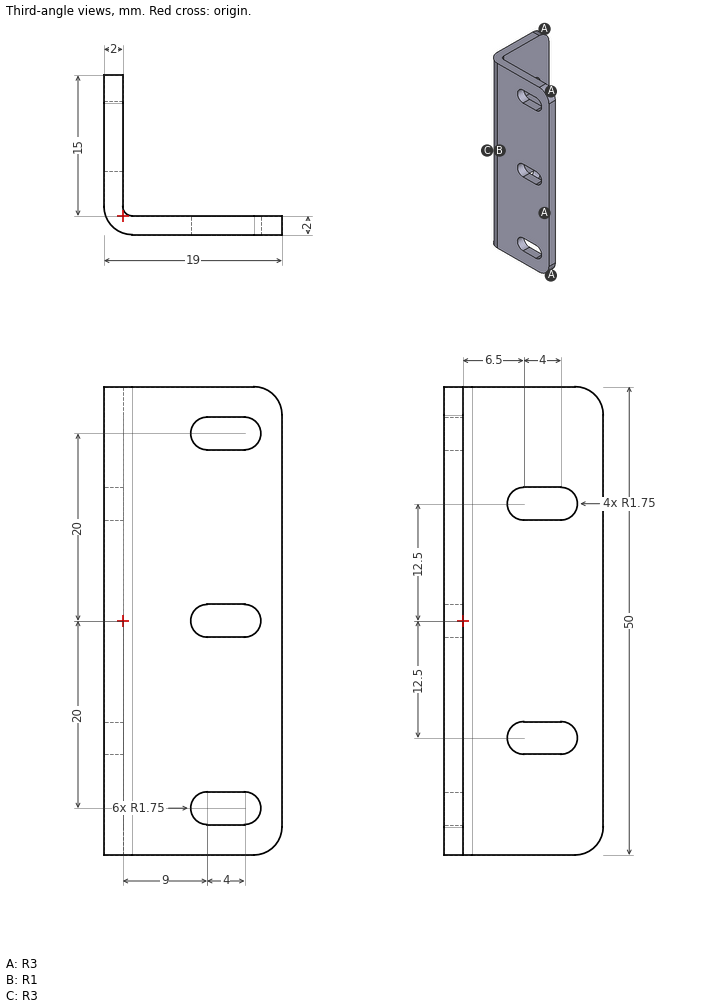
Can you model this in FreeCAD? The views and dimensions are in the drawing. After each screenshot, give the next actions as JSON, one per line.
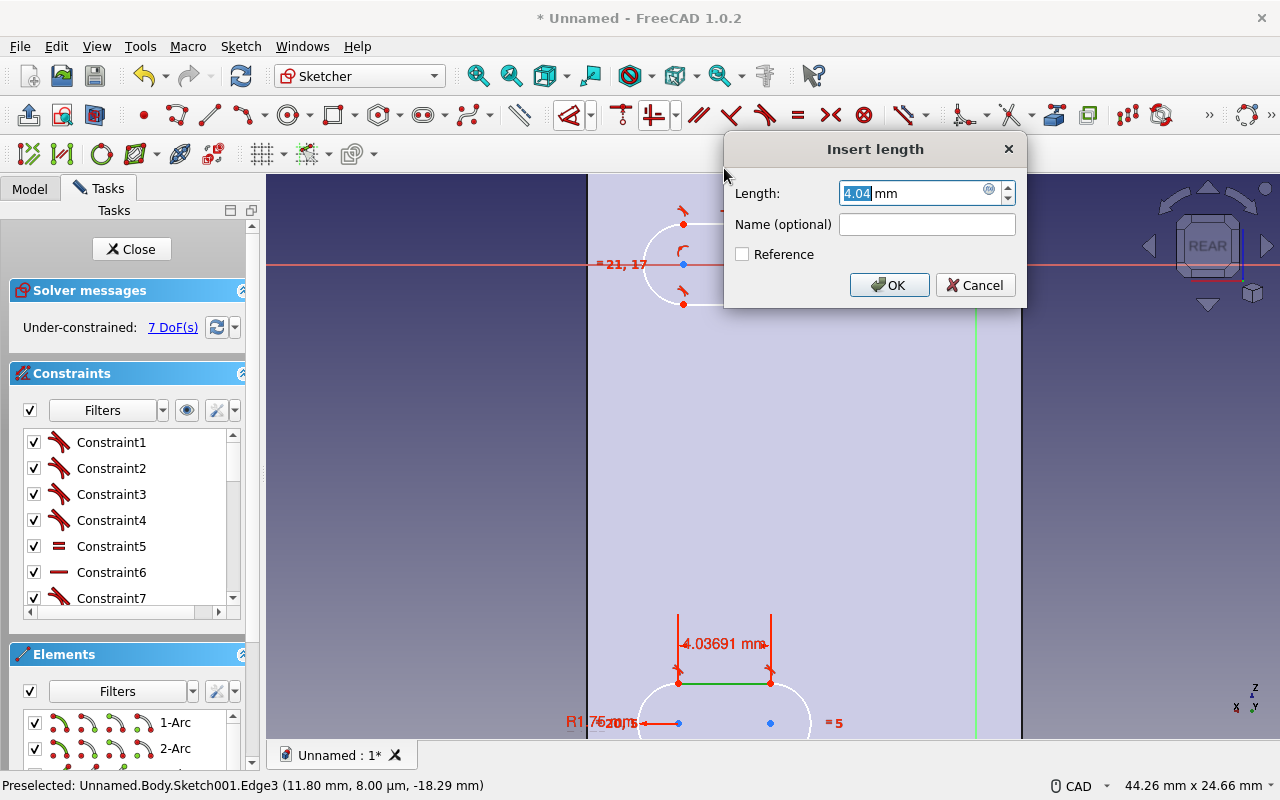
{"action": "type", "text": "4"}
{"action": "key", "text": "Return"}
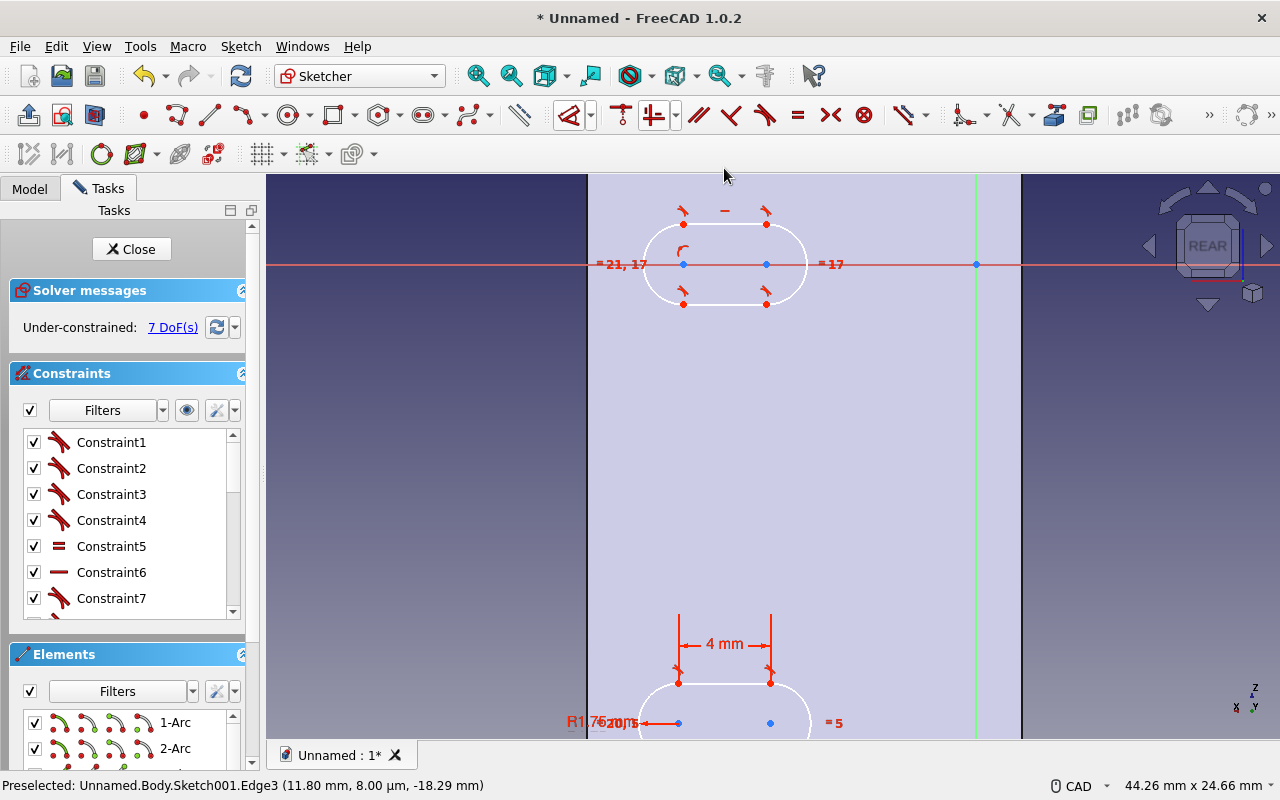
{"action": "scroll", "coordinate": [645, 568], "scroll_direction": "down", "scroll_amount": 5}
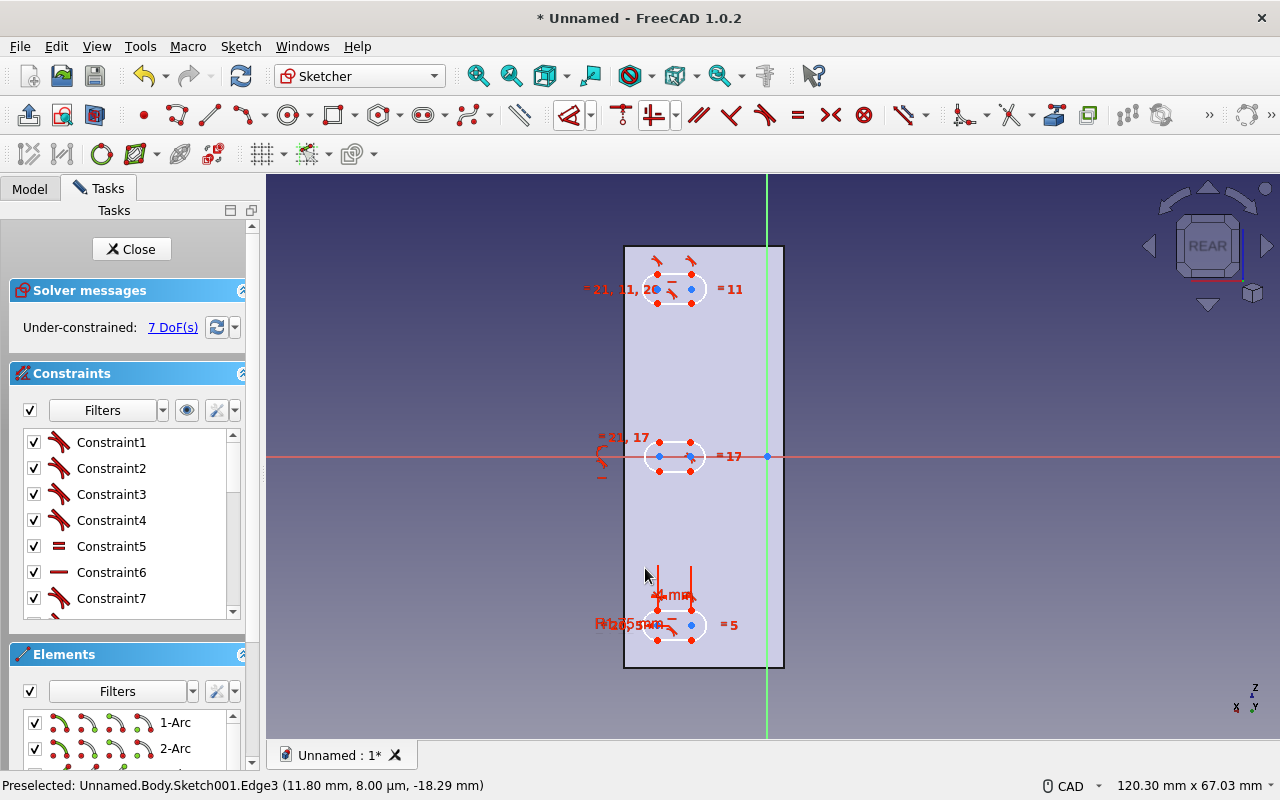
{"action": "scroll", "coordinate": [668, 274], "scroll_direction": "up", "scroll_amount": 2}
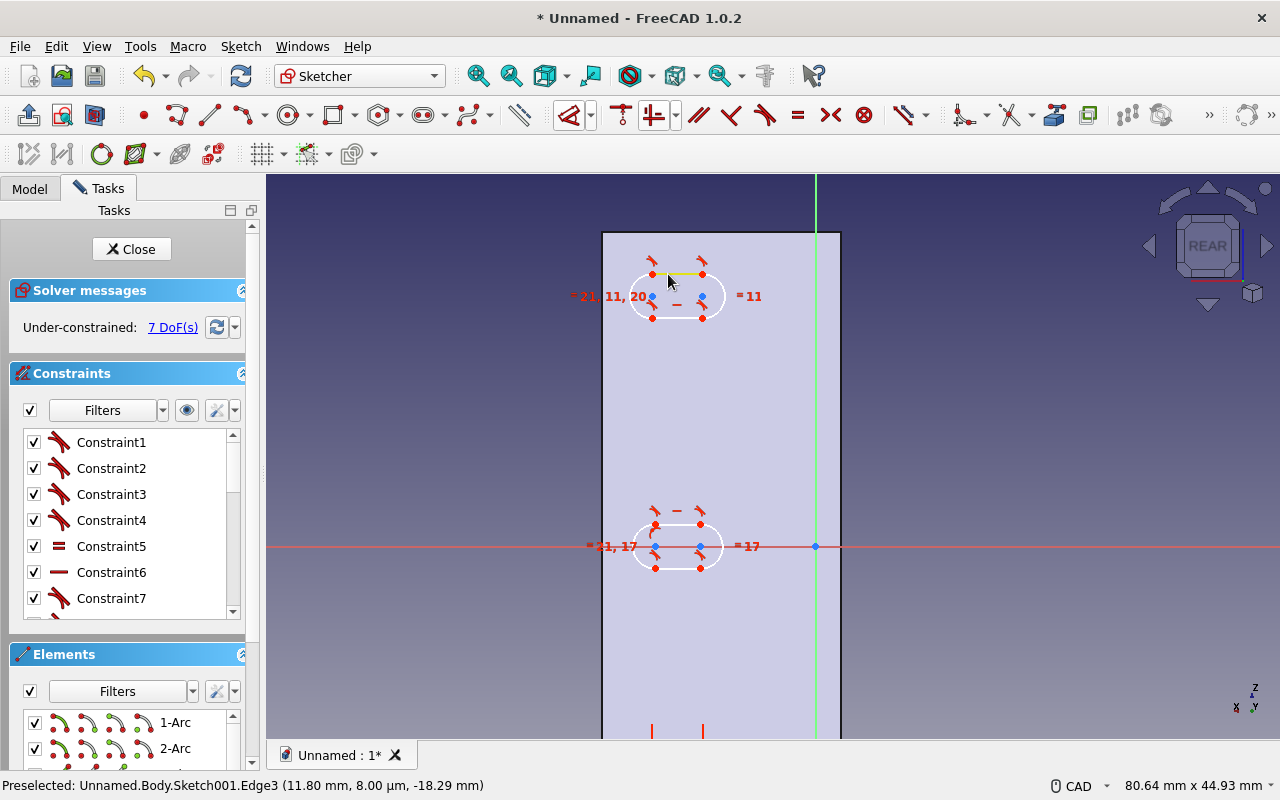
{"action": "left_click", "coordinate": [667, 274]}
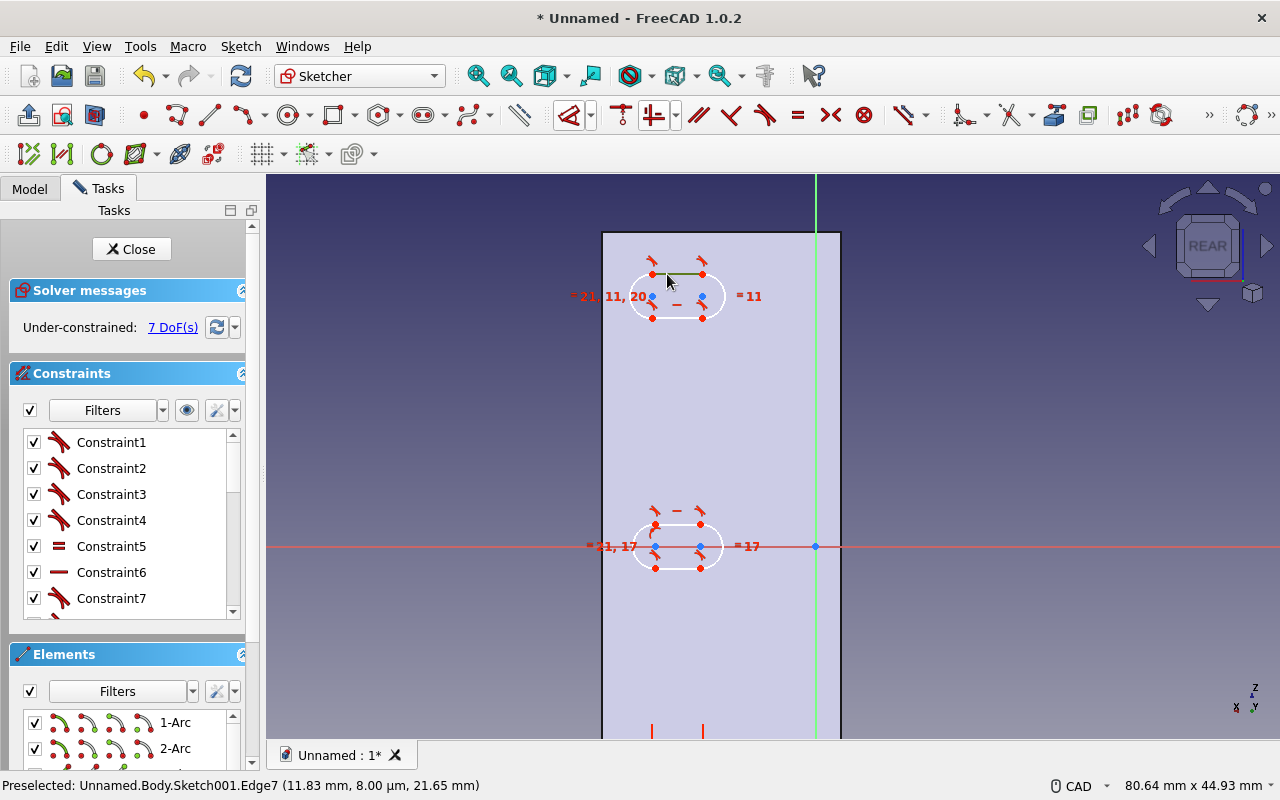
{"action": "key", "text": "l"}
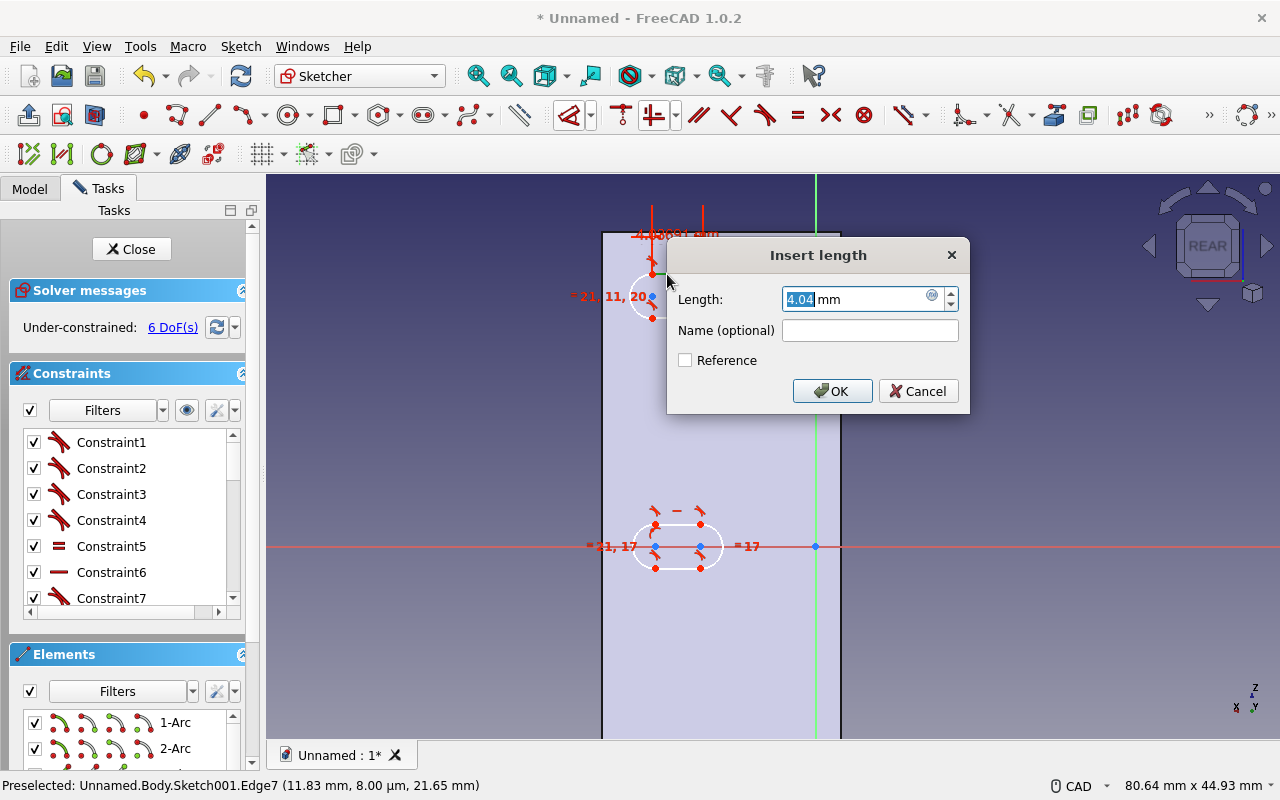
{"action": "type", "text": "4"}
{"action": "key", "text": "Return"}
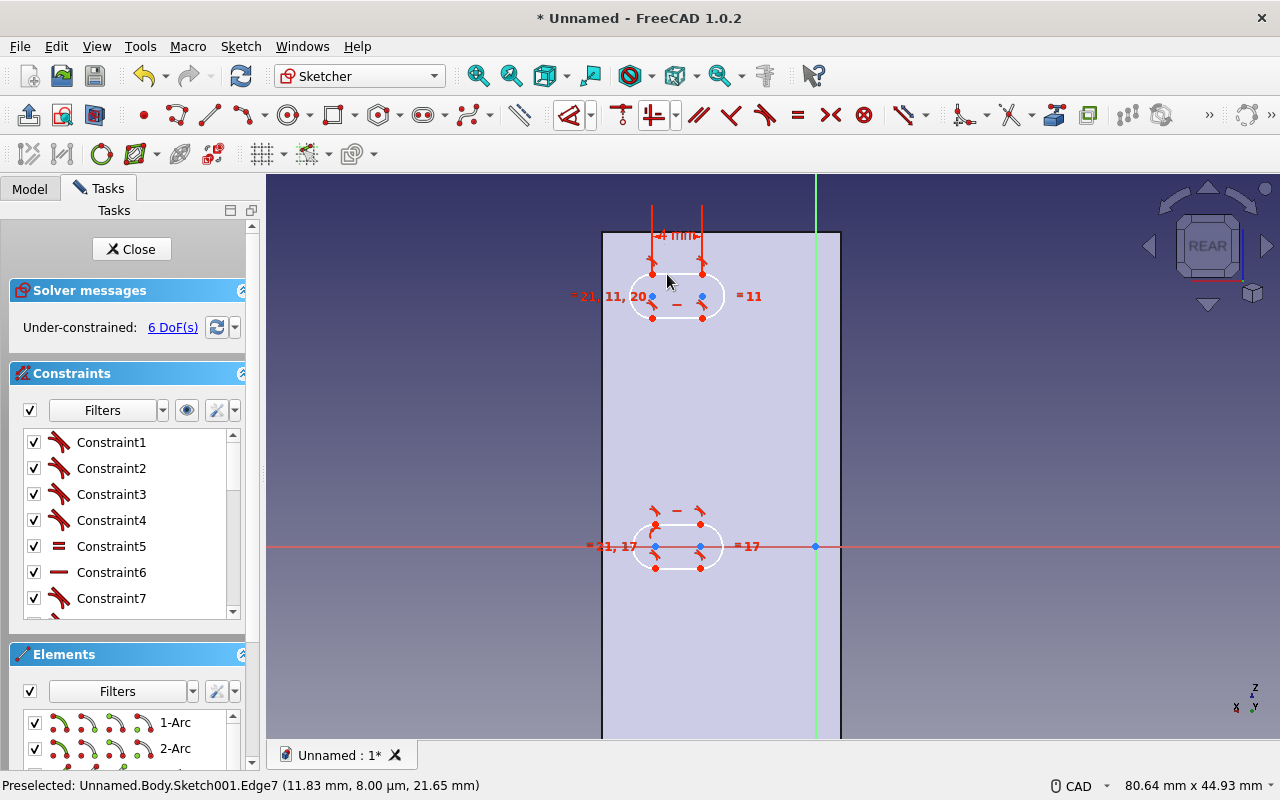
{"action": "left_click", "coordinate": [669, 525]}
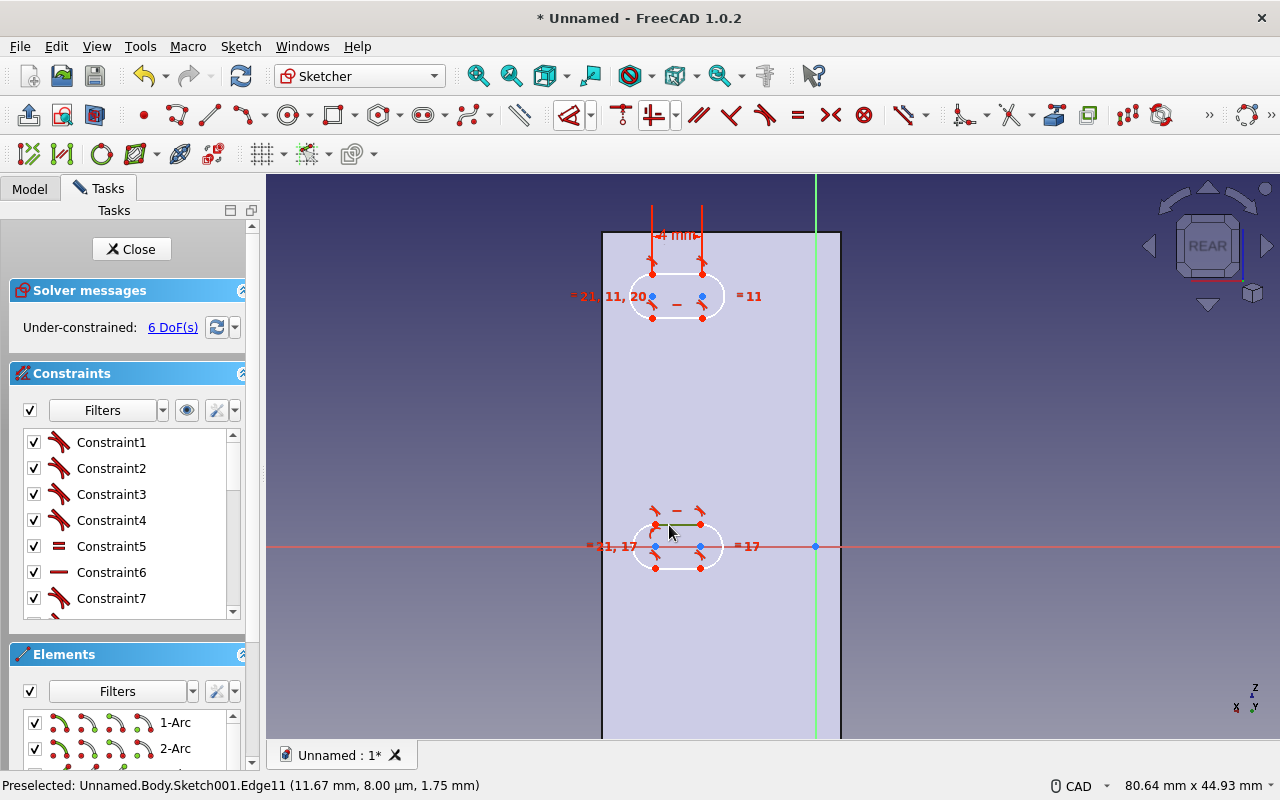
{"action": "key", "text": "l"}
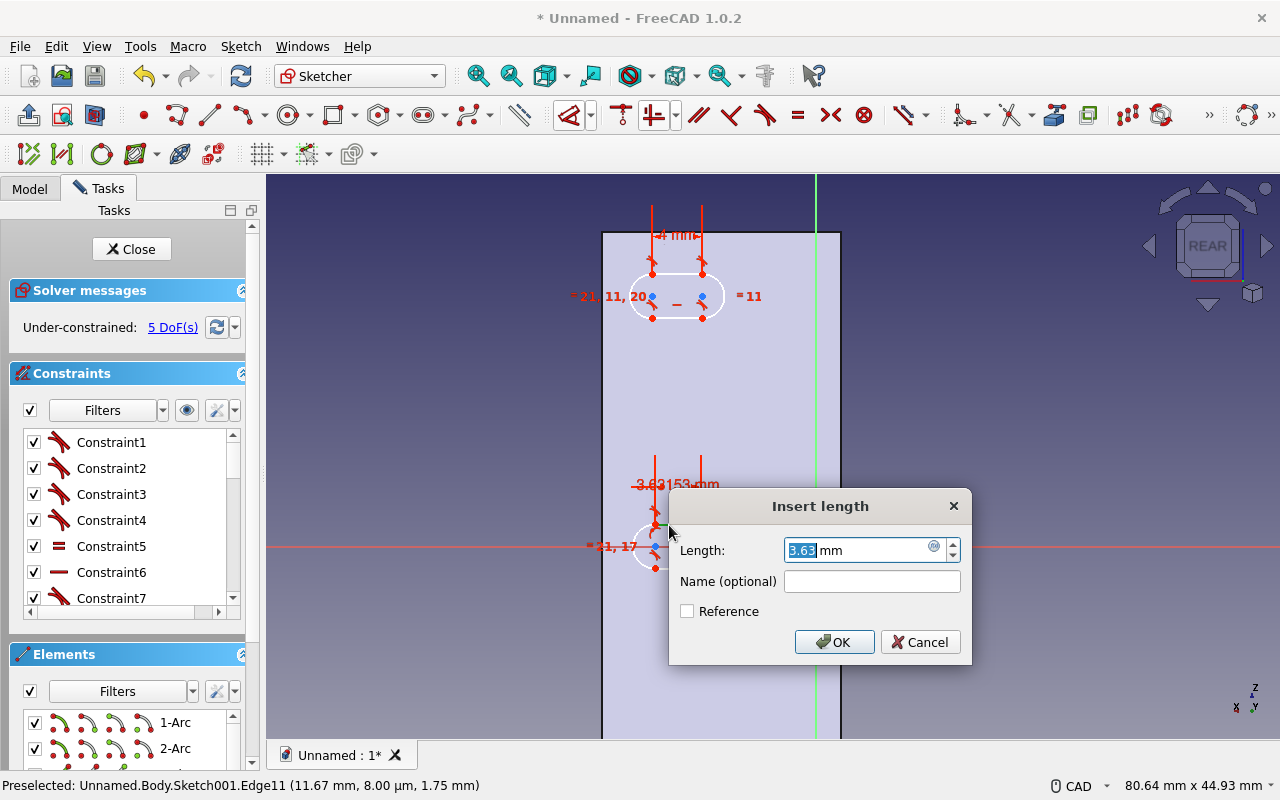
{"action": "type", "text": "4"}
{"action": "key", "text": "Return"}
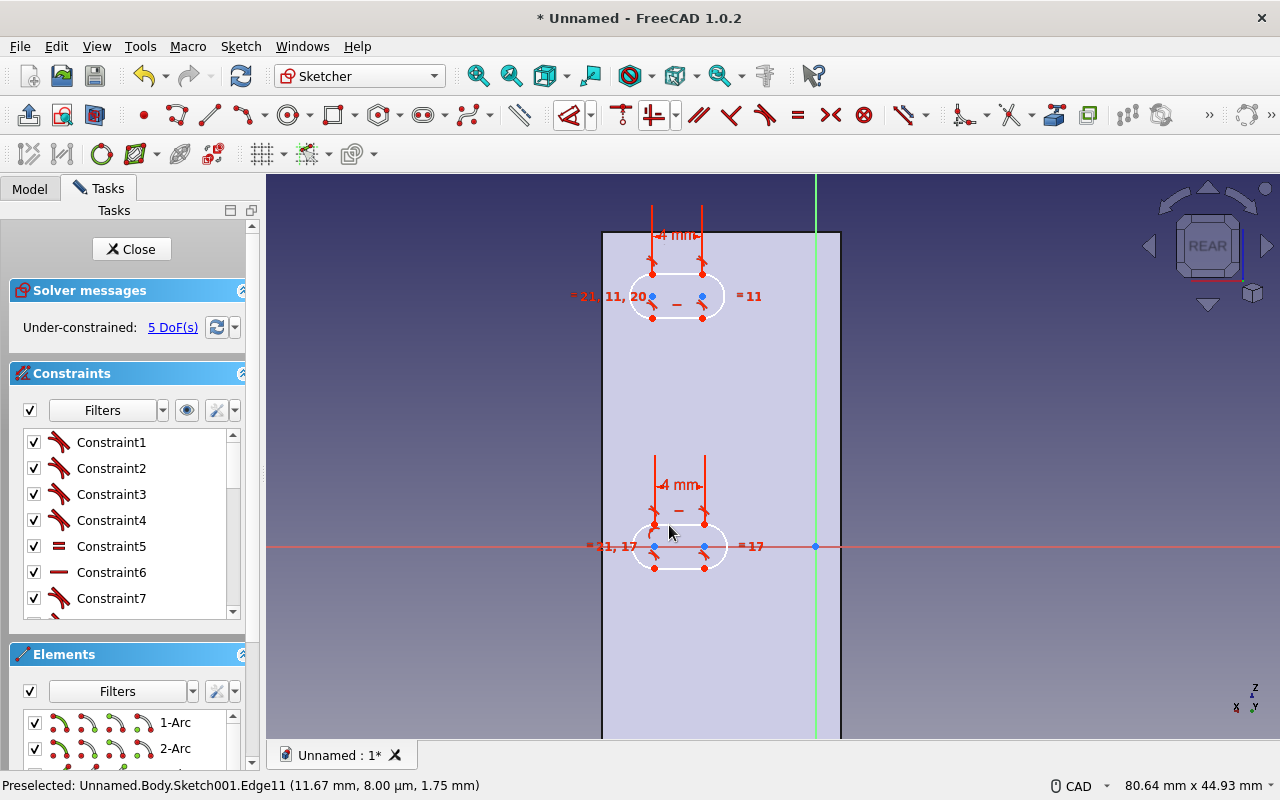
{"action": "scroll", "coordinate": [667, 273], "scroll_direction": "down", "scroll_amount": 2}